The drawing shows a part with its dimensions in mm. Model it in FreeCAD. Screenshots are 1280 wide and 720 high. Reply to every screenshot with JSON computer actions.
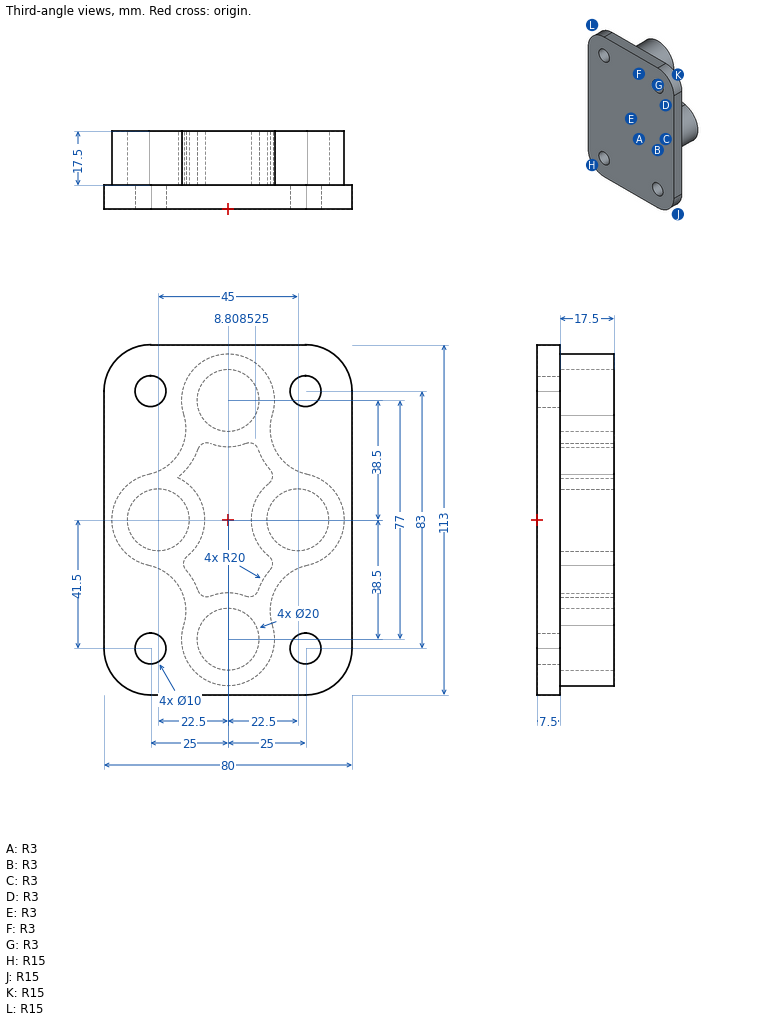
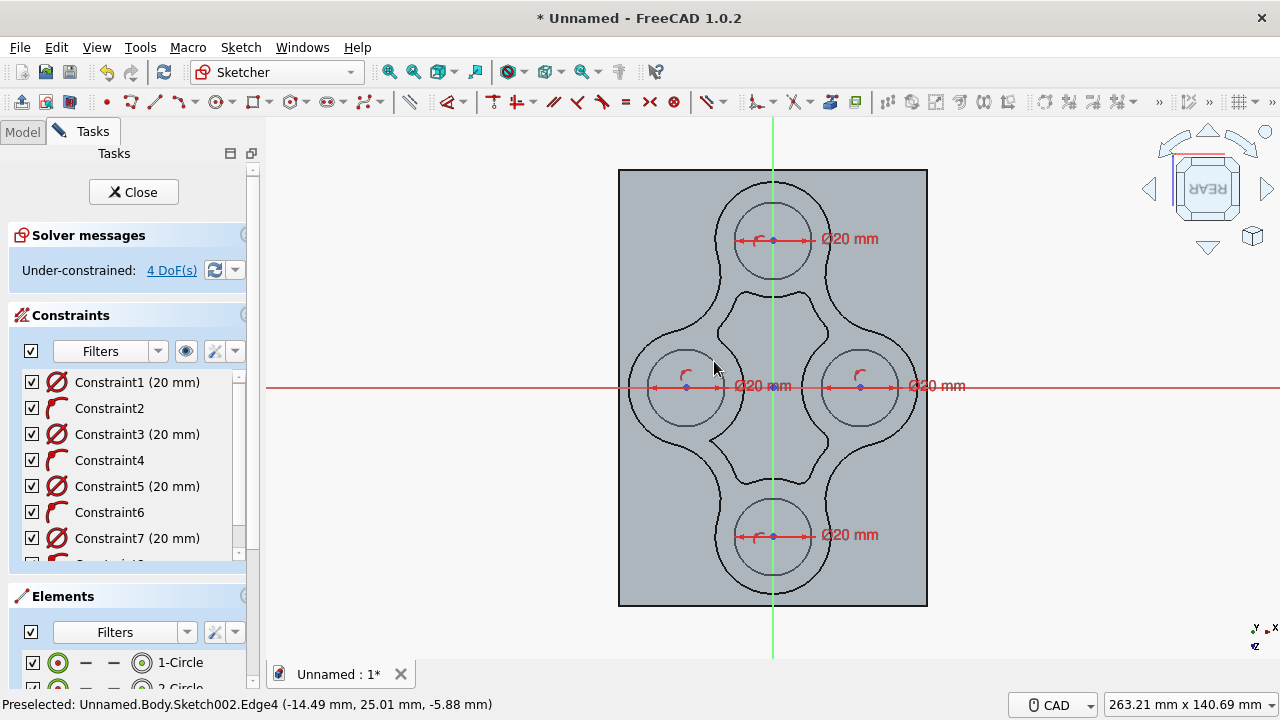
{"action": "key", "text": "d"}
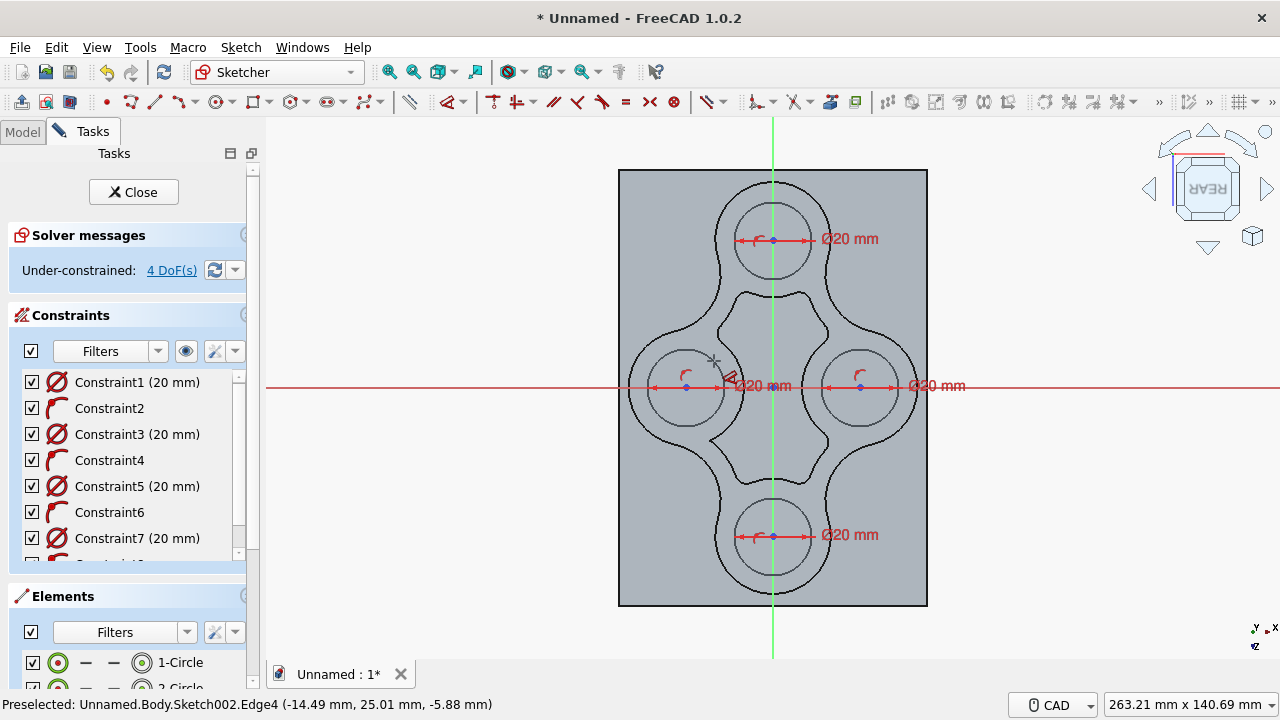
{"action": "left_click", "coordinate": [773, 241]}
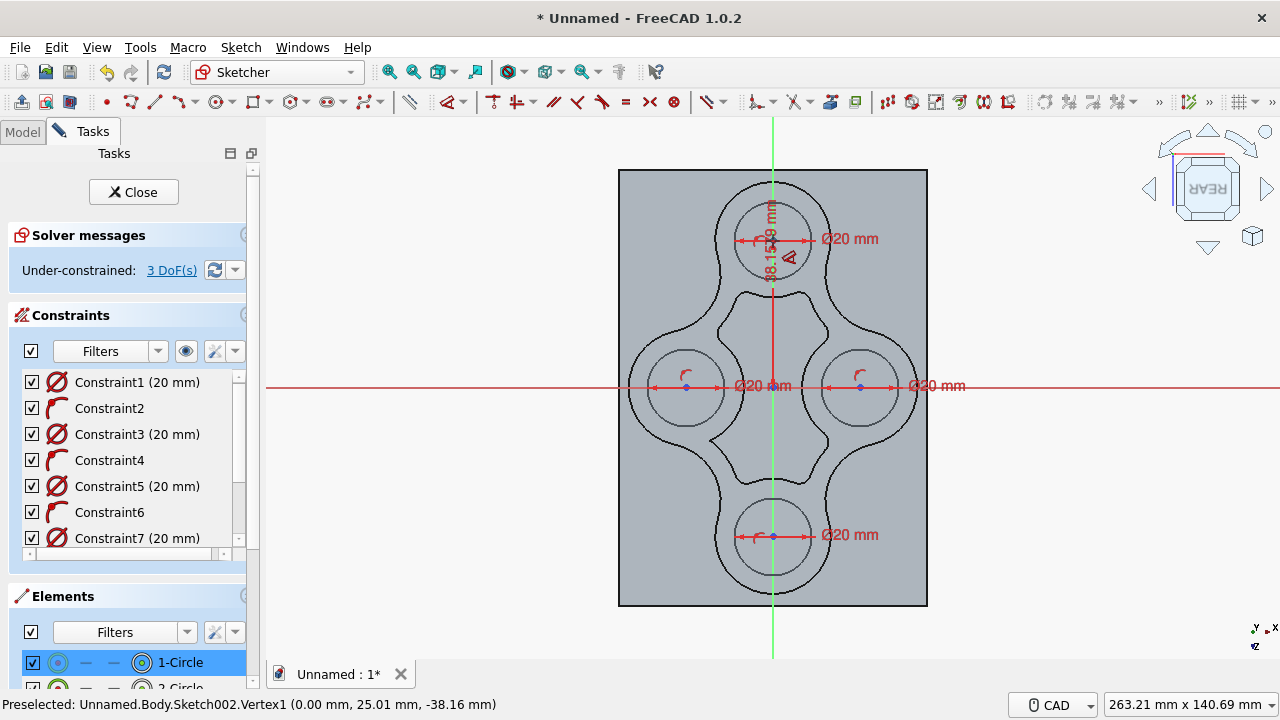
{"action": "left_click", "coordinate": [773, 537]}
{"action": "left_click", "coordinate": [807, 321]}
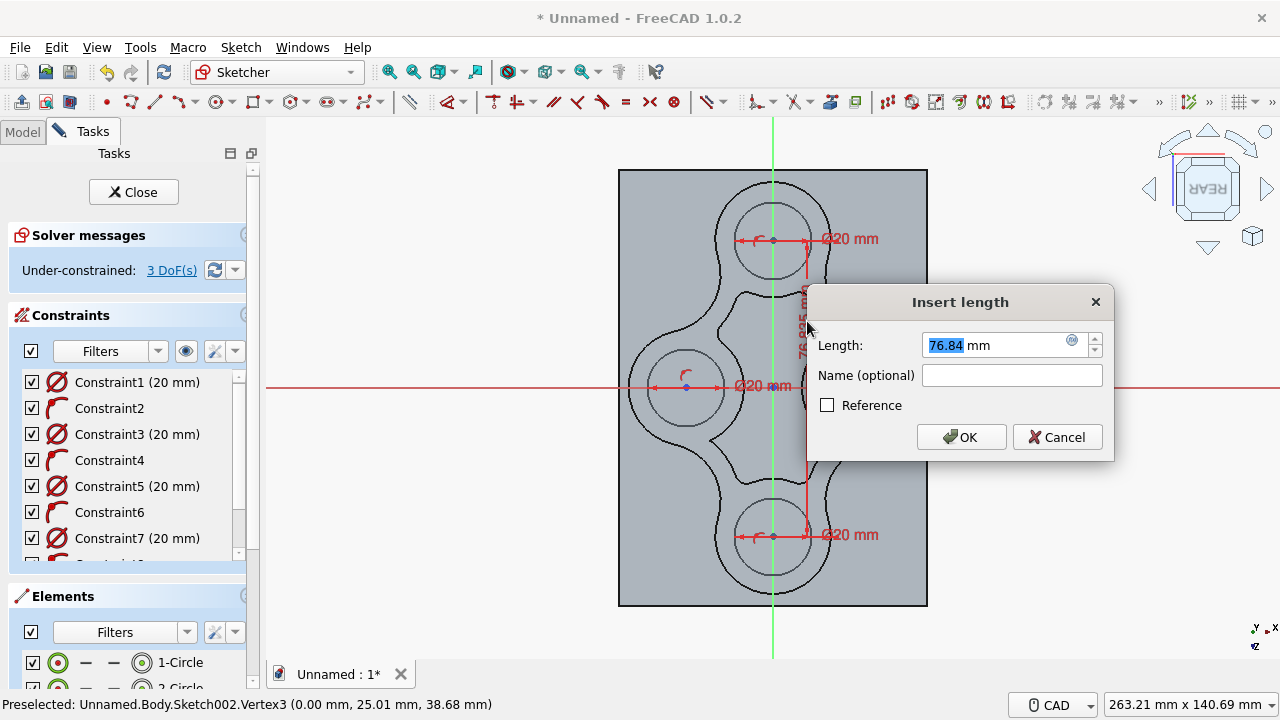
{"action": "type", "text": "77"}
{"action": "key", "text": "Return"}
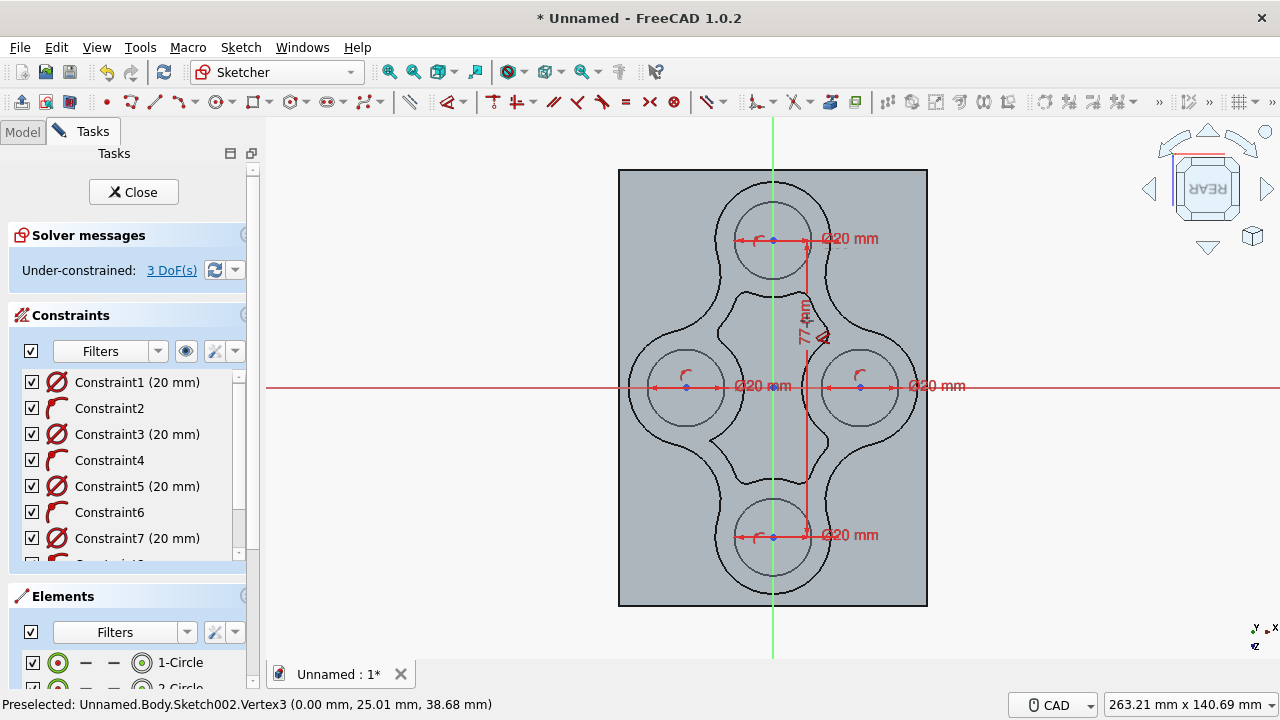
{"action": "left_click", "coordinate": [860, 388]}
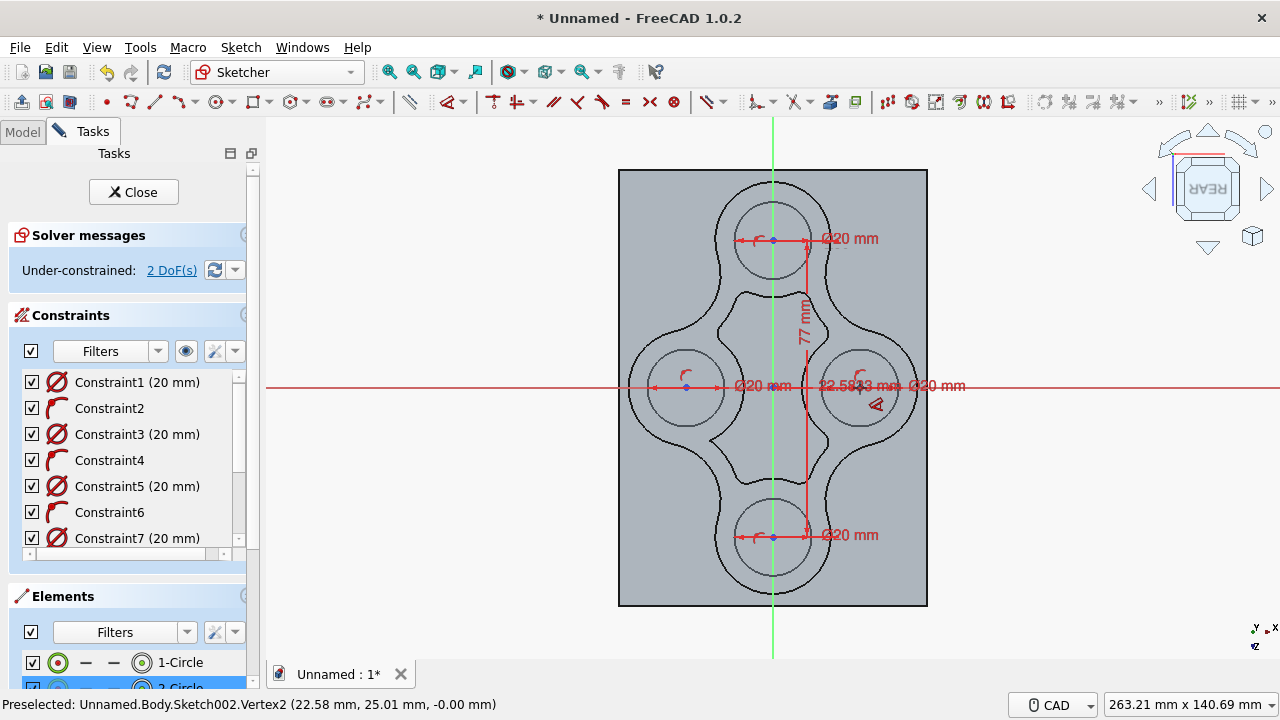
{"action": "left_click", "coordinate": [686, 388]}
{"action": "left_click", "coordinate": [733, 422]}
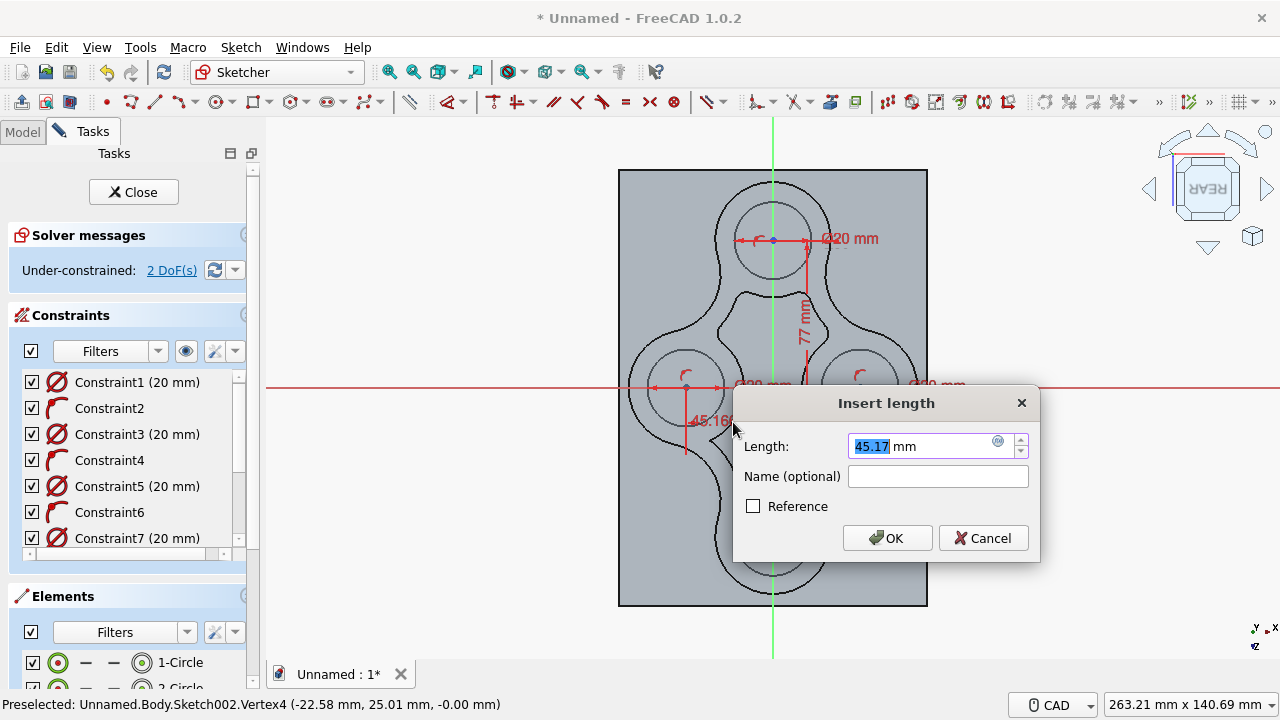
{"action": "type", "text": "45"}
{"action": "key", "text": "Return"}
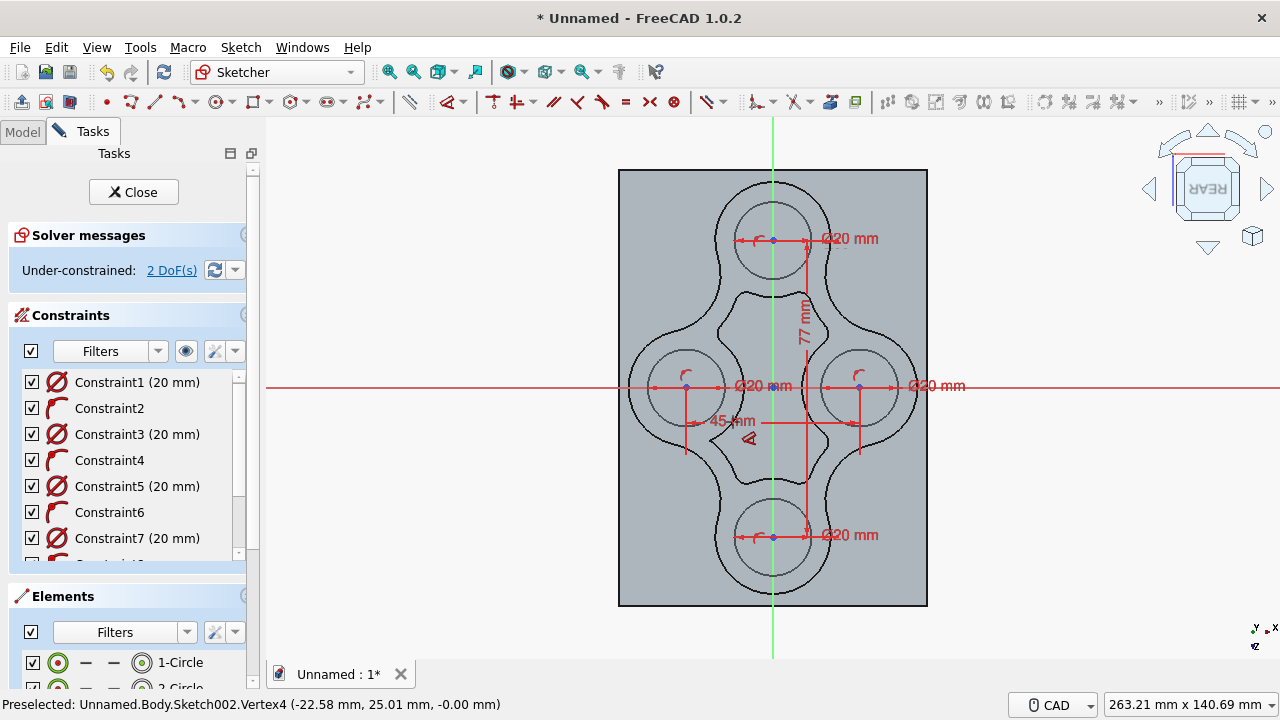
{"action": "left_click", "coordinate": [773, 241]}
{"action": "left_click", "coordinate": [807, 280]}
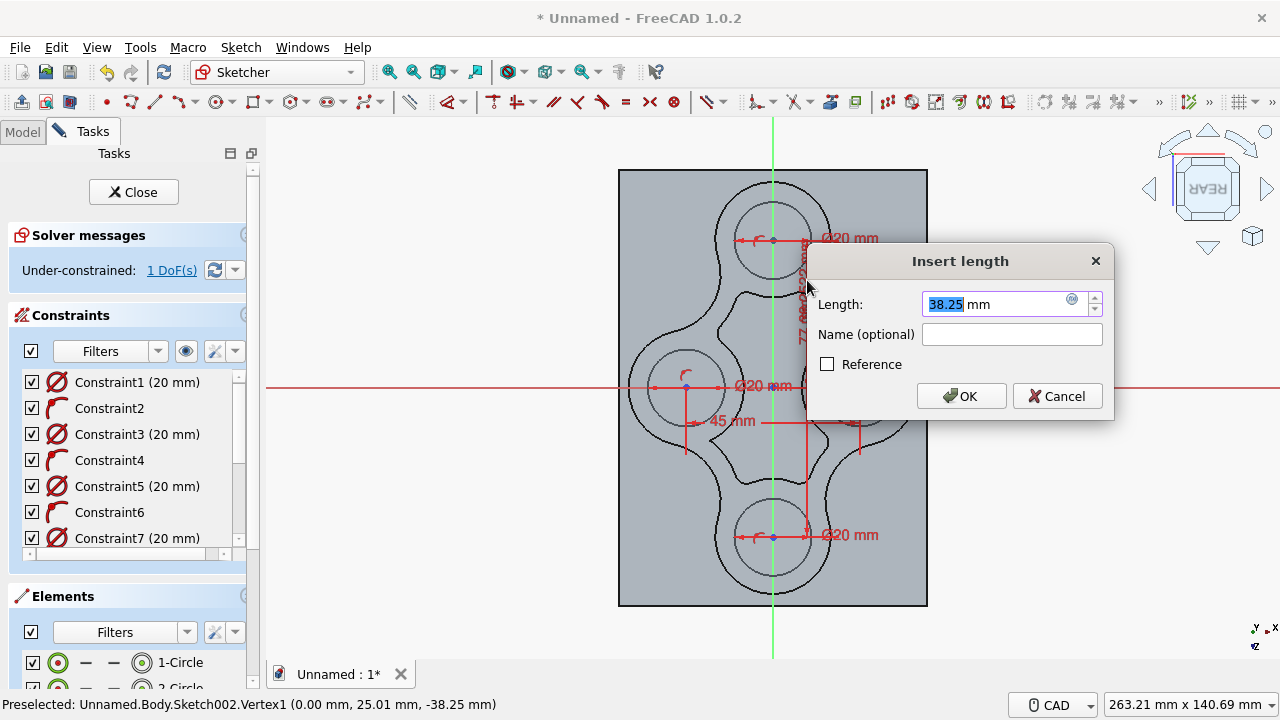
{"action": "type", "text": "38.5"}
{"action": "key", "text": "Return"}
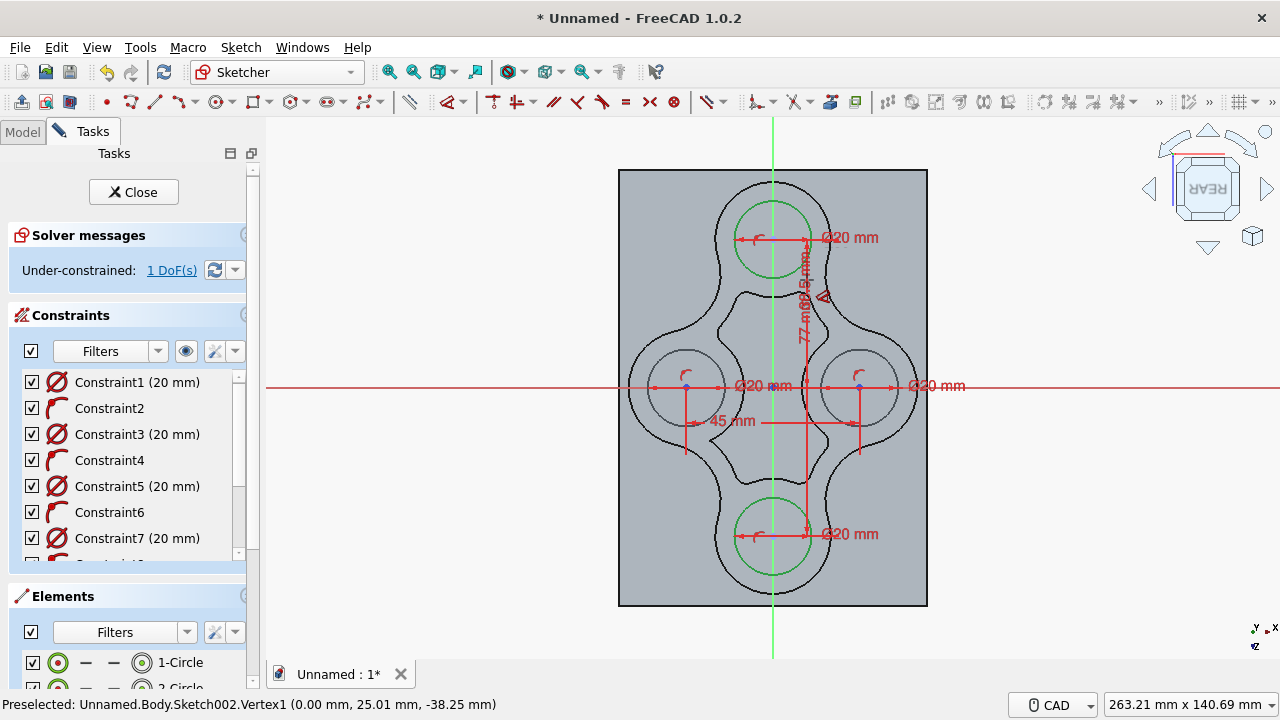
{"action": "left_click", "coordinate": [860, 388]}
{"action": "left_click", "coordinate": [816, 422]}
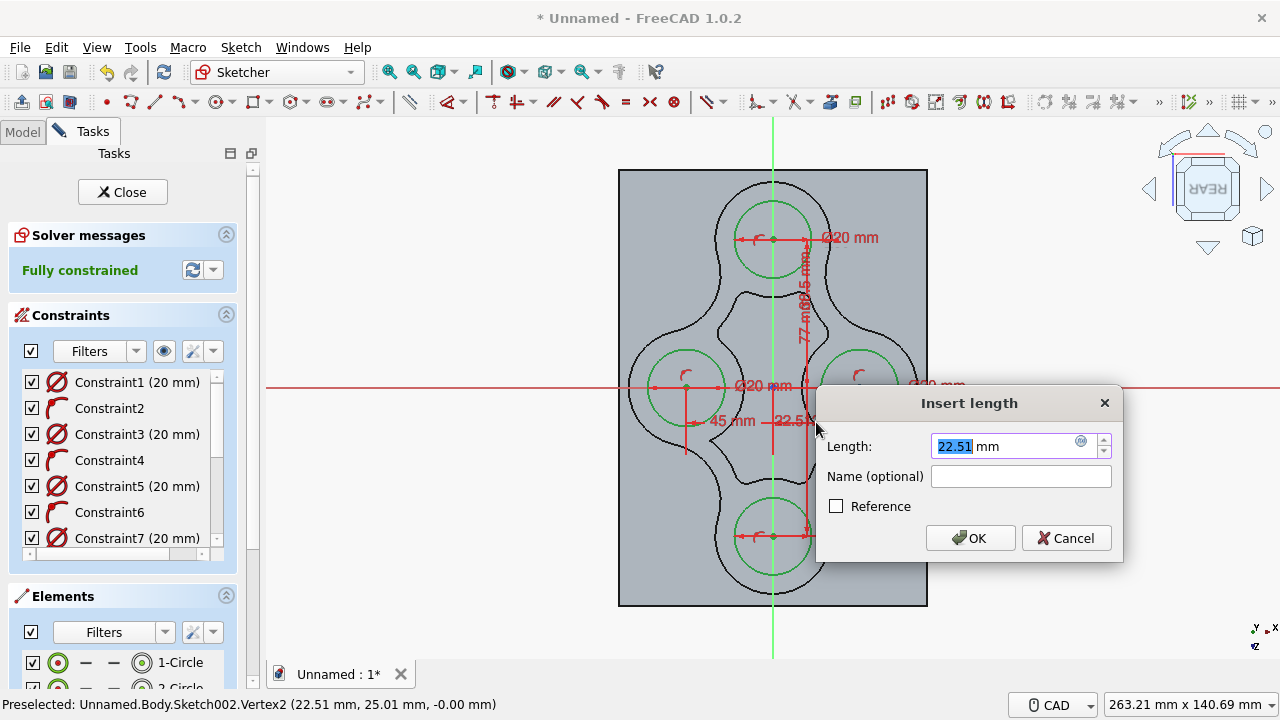
{"action": "type", "text": "22.5"}
{"action": "key", "text": "Return"}
{"action": "key", "text": "Escape"}